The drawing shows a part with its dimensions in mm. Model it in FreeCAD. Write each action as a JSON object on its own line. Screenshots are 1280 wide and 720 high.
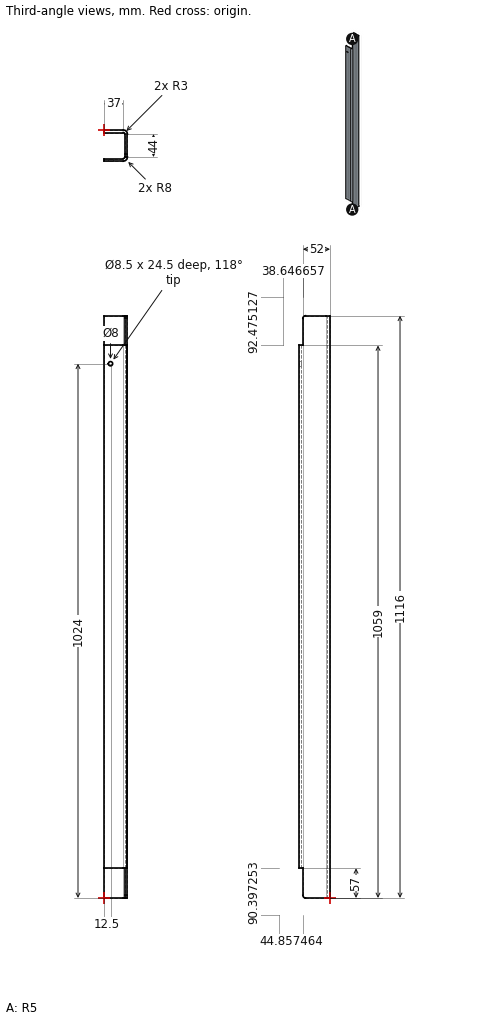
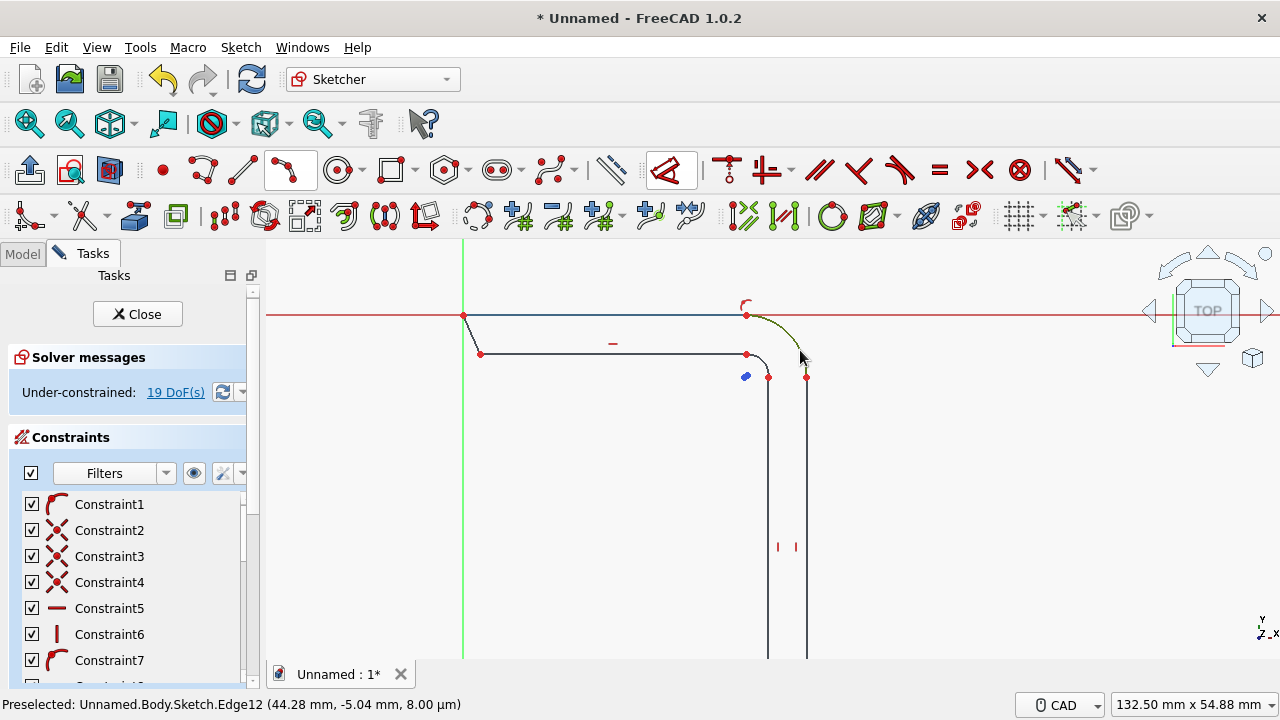
{"action": "key", "text": "t"}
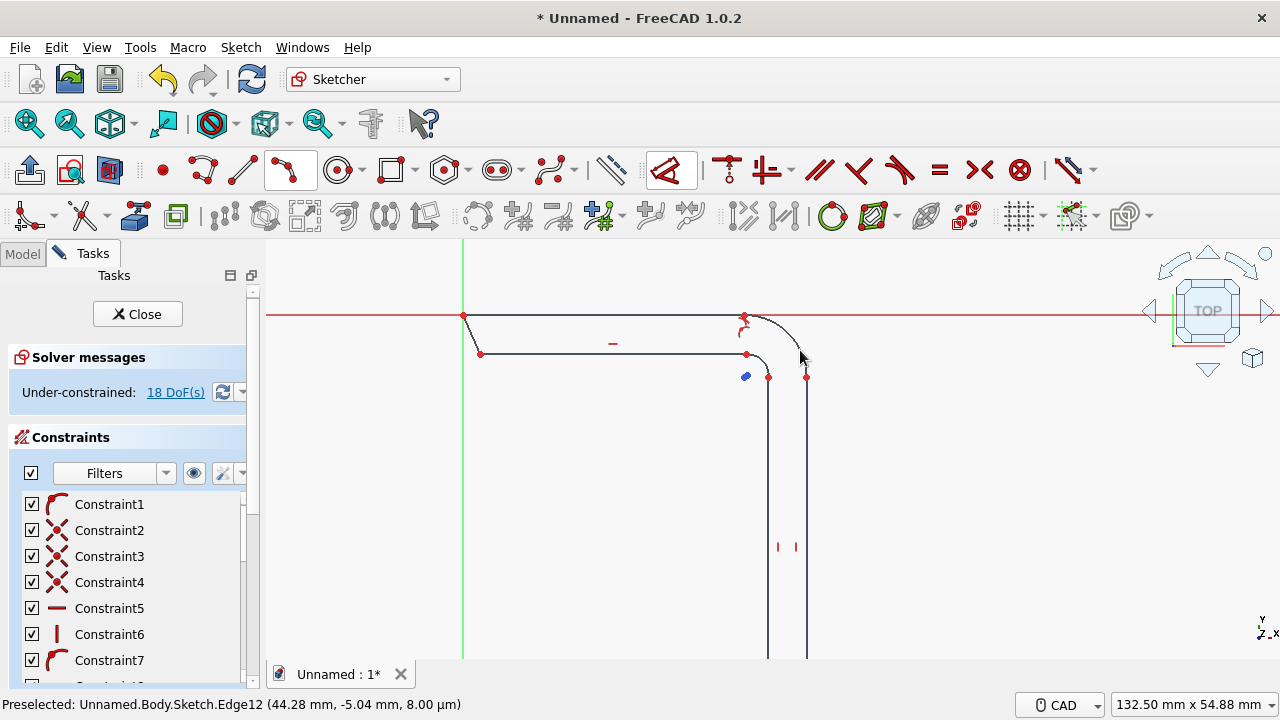
{"action": "left_click", "coordinate": [560, 354]}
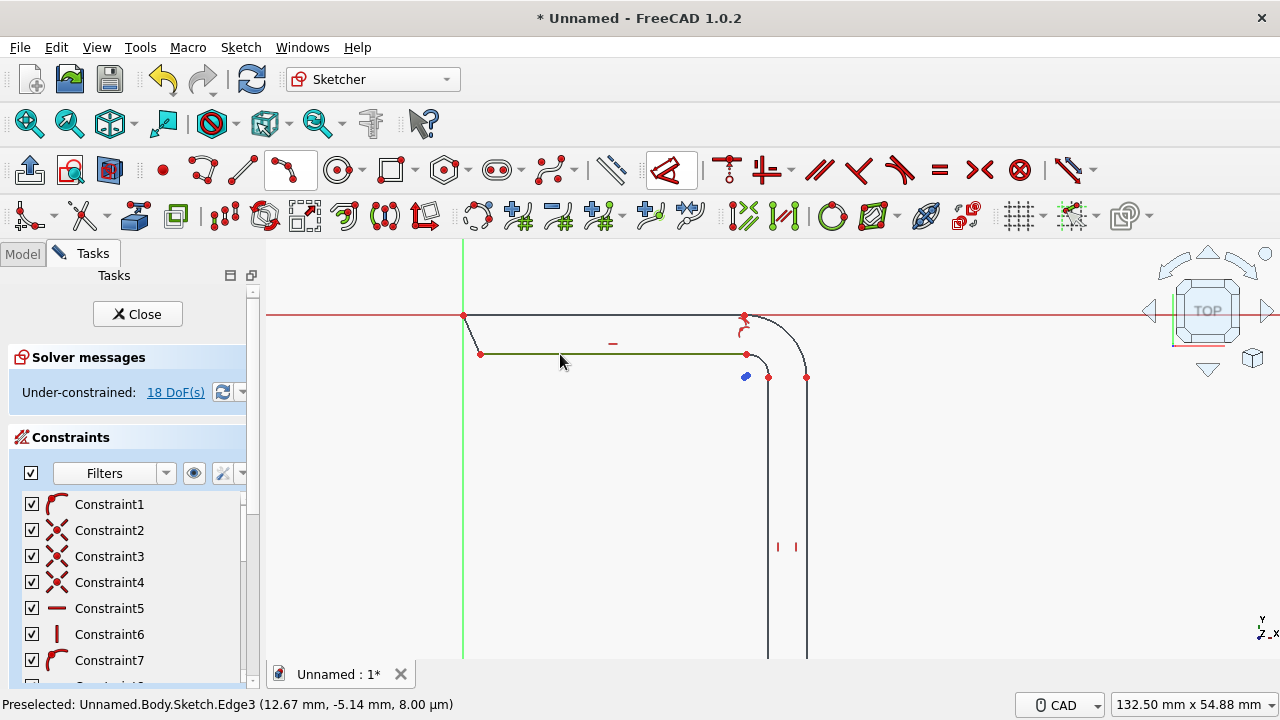
{"action": "scroll", "coordinate": [767, 367], "scroll_direction": "up", "scroll_amount": 2}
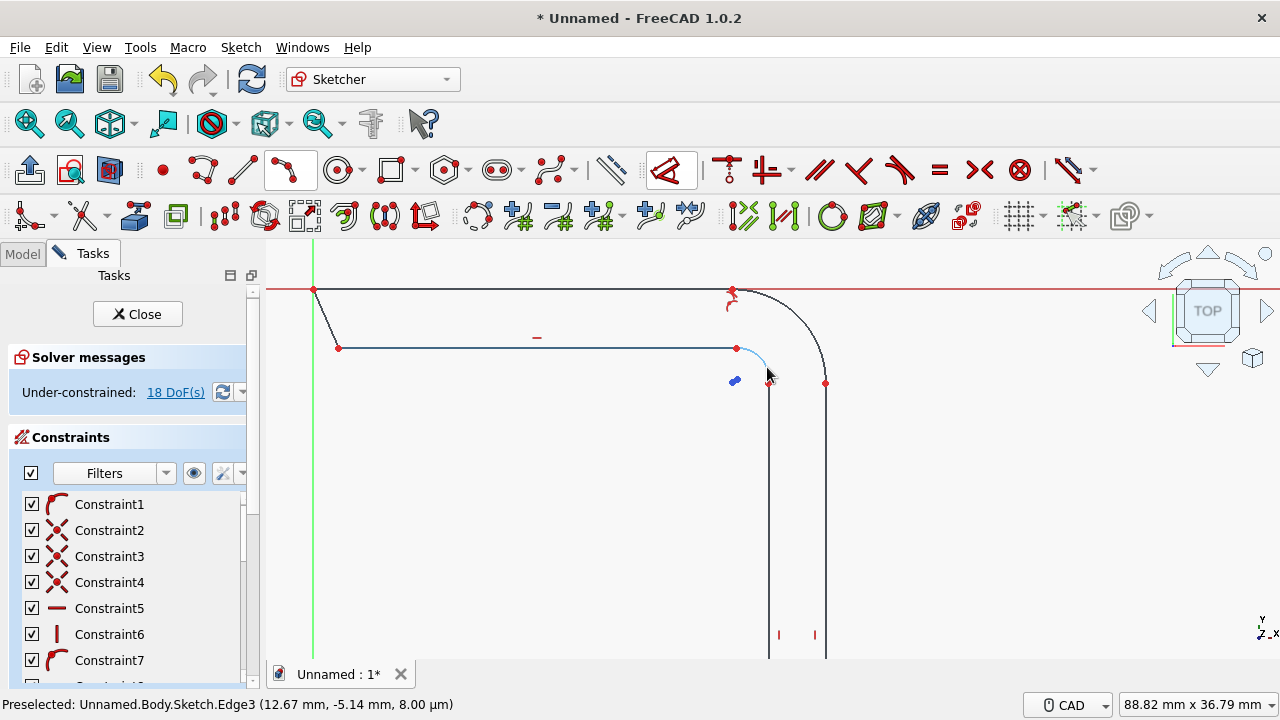
{"action": "left_click", "coordinate": [767, 367]}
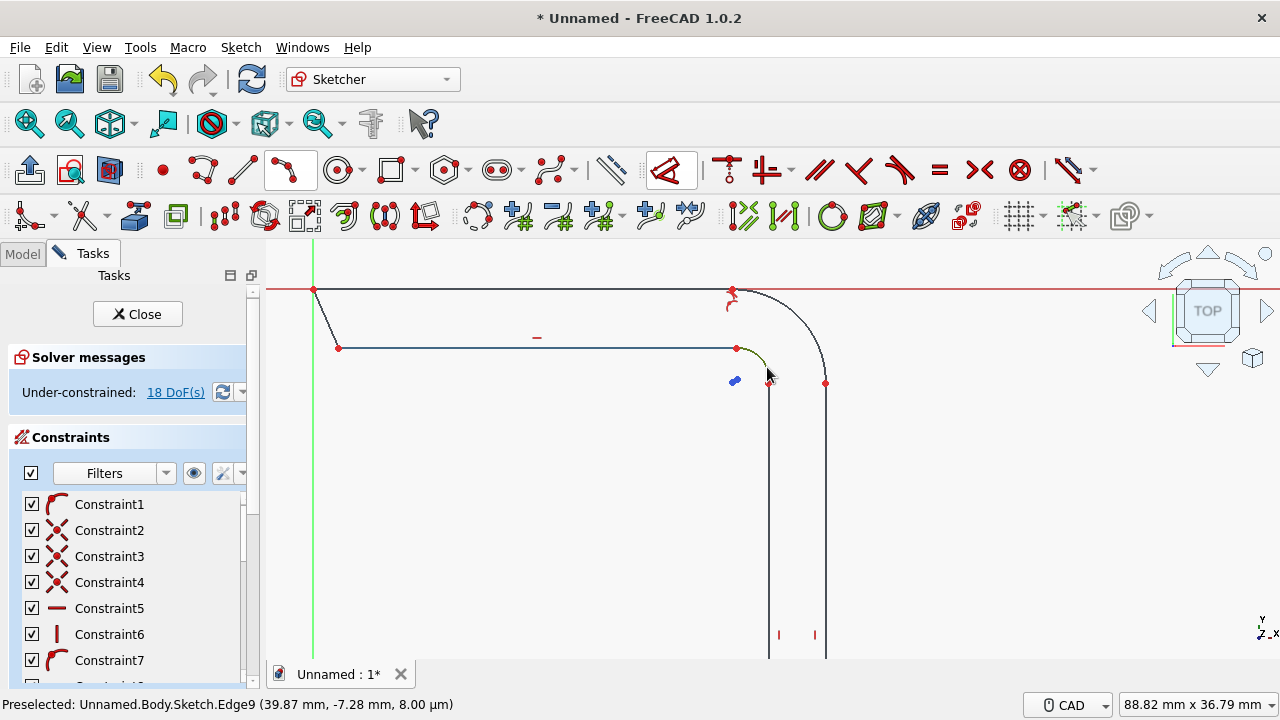
{"action": "left_click", "coordinate": [900, 170]}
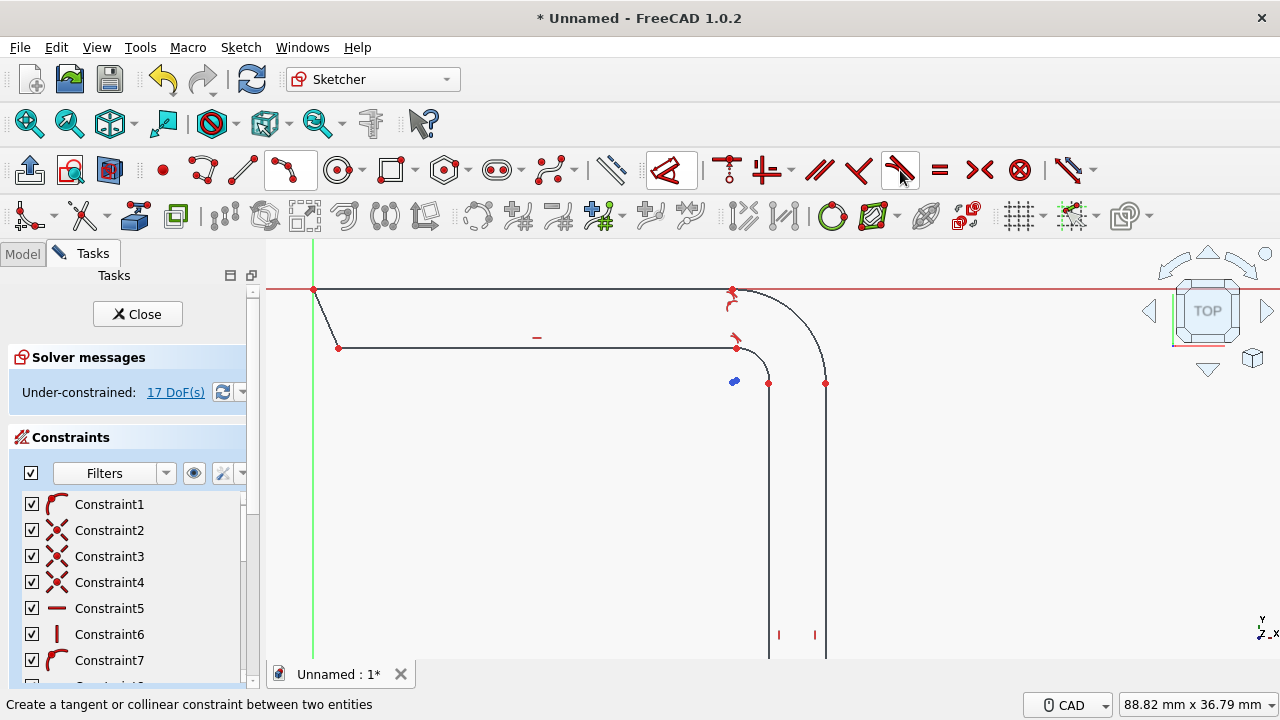
{"action": "left_click", "coordinate": [769, 534]}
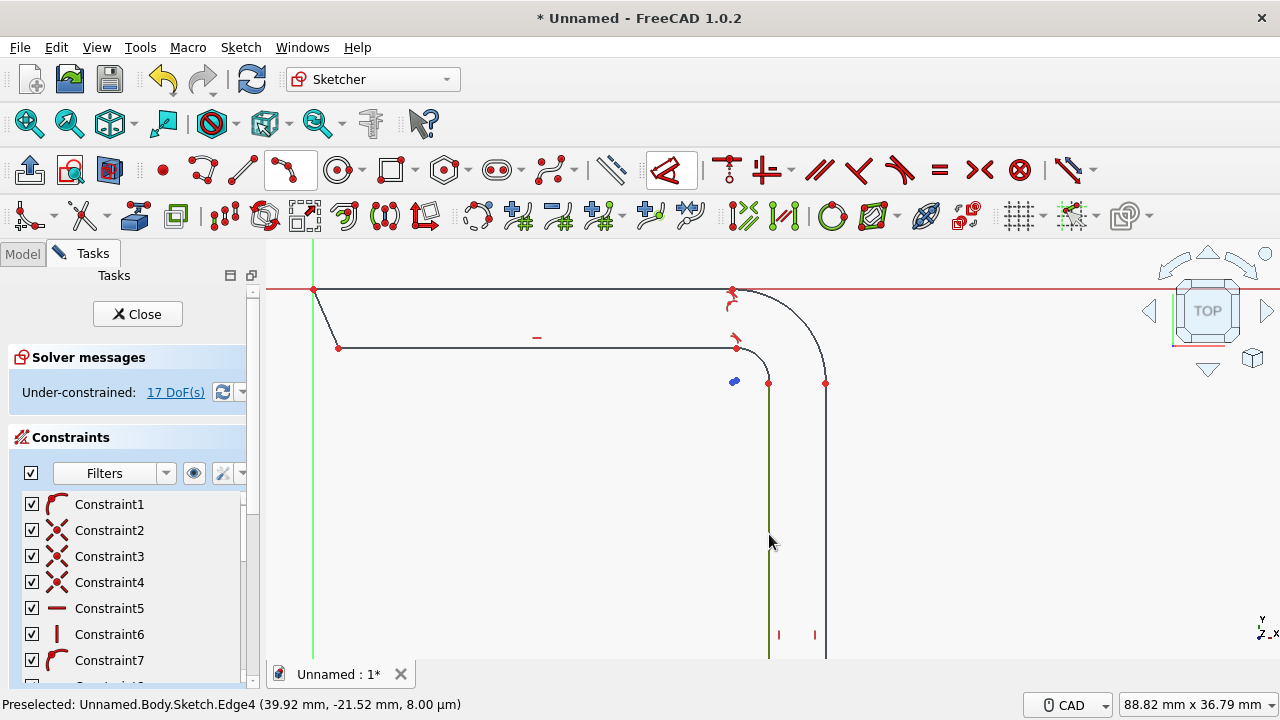
{"action": "left_click", "coordinate": [766, 367]}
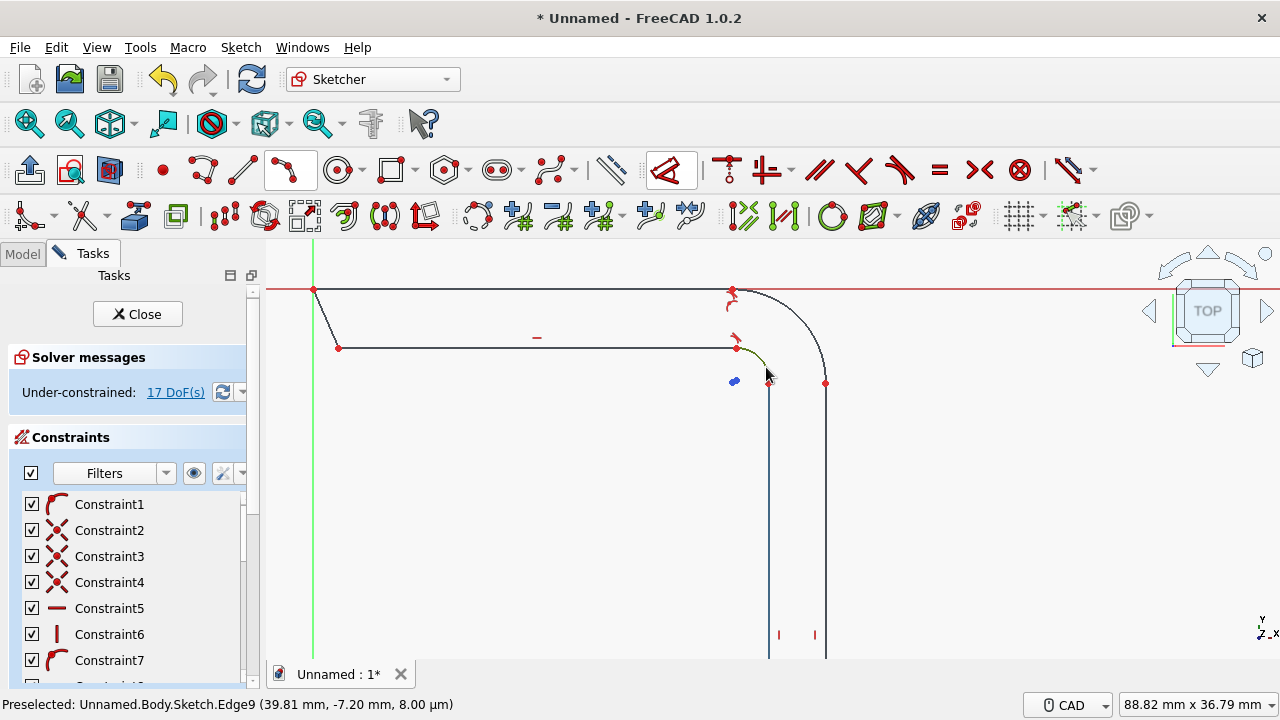
{"action": "key", "text": "t"}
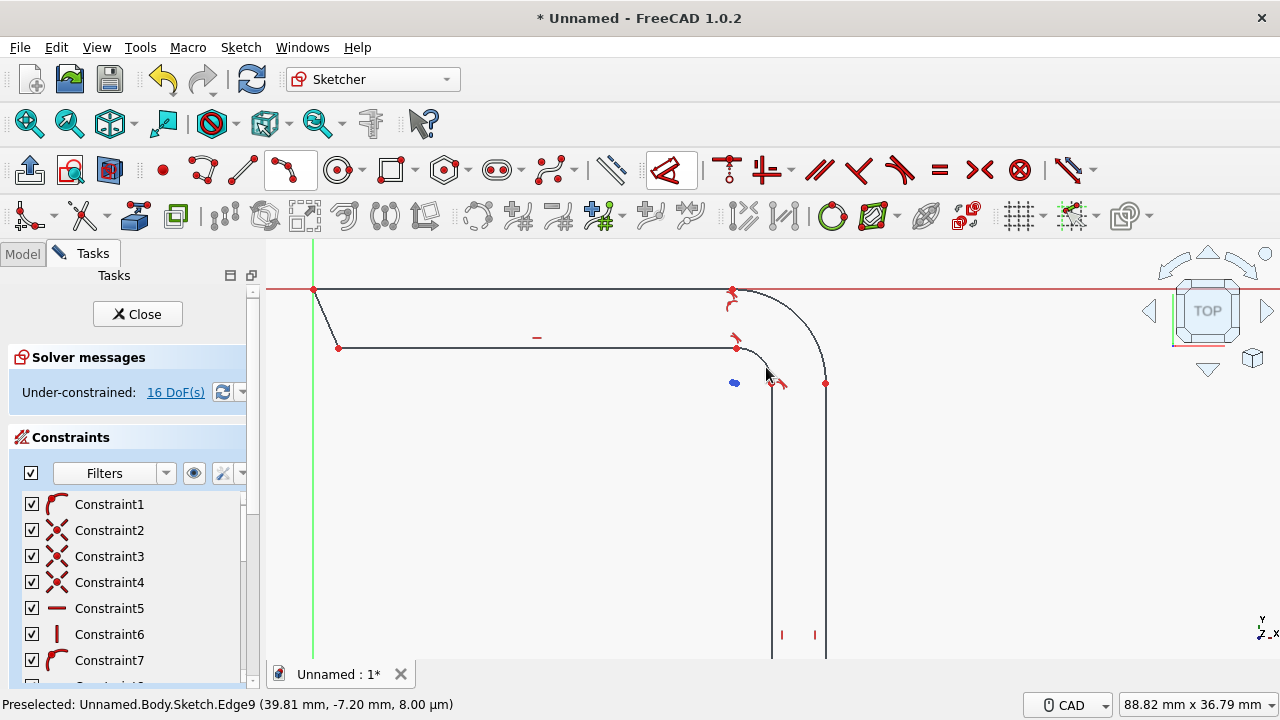
{"action": "left_click", "coordinate": [772, 534]}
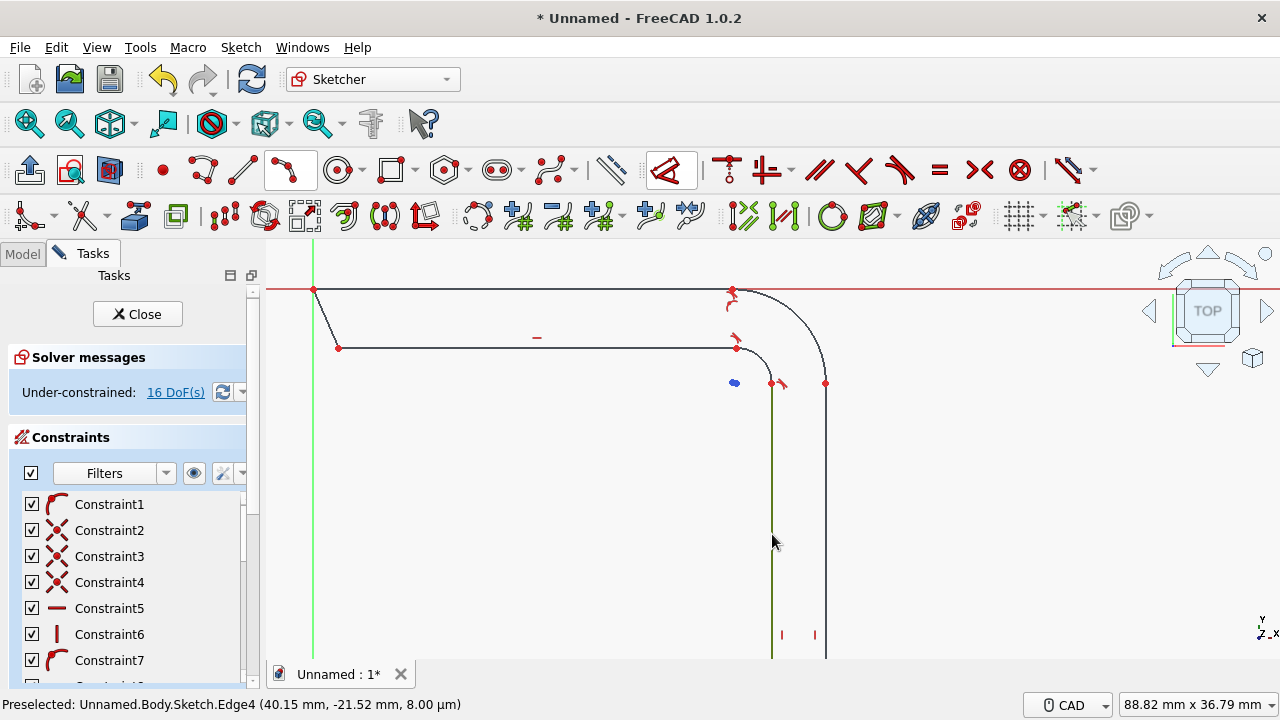
{"action": "scroll", "coordinate": [783, 343], "scroll_direction": "down", "scroll_amount": 5}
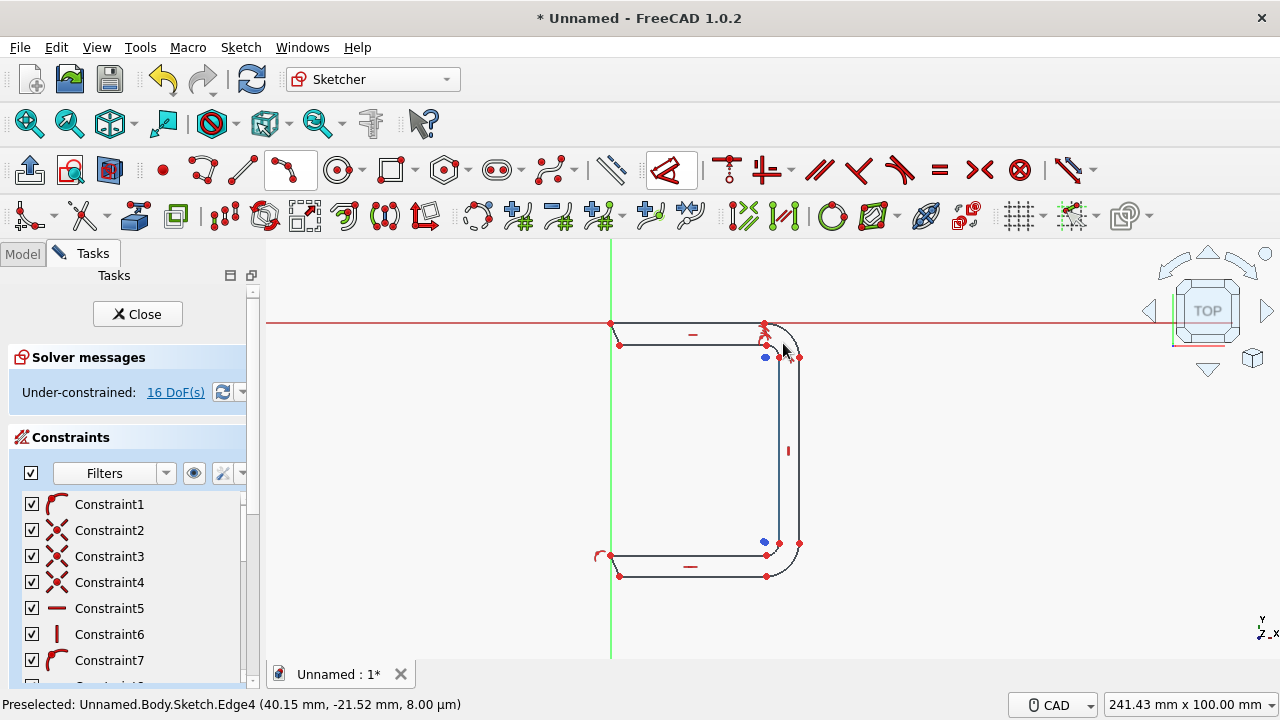
{"action": "scroll", "coordinate": [772, 554], "scroll_direction": "up", "scroll_amount": 5}